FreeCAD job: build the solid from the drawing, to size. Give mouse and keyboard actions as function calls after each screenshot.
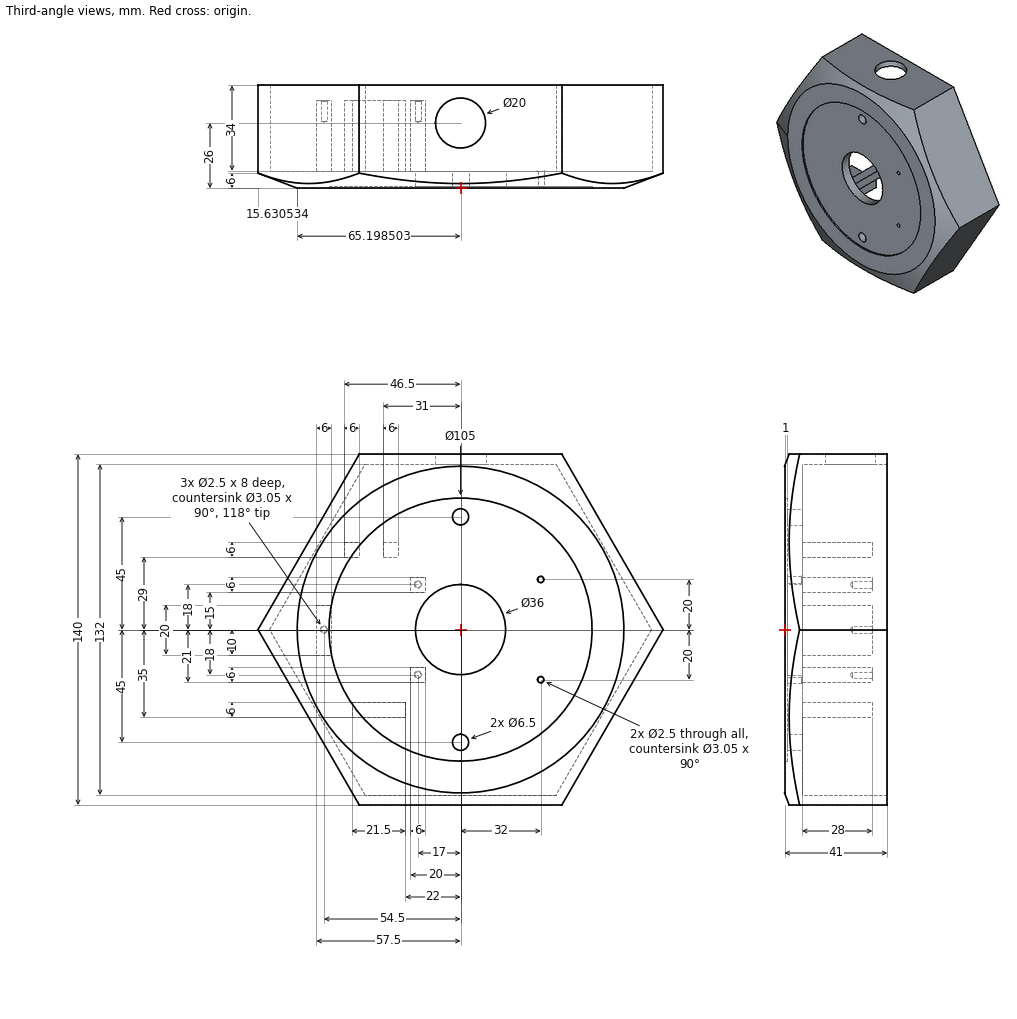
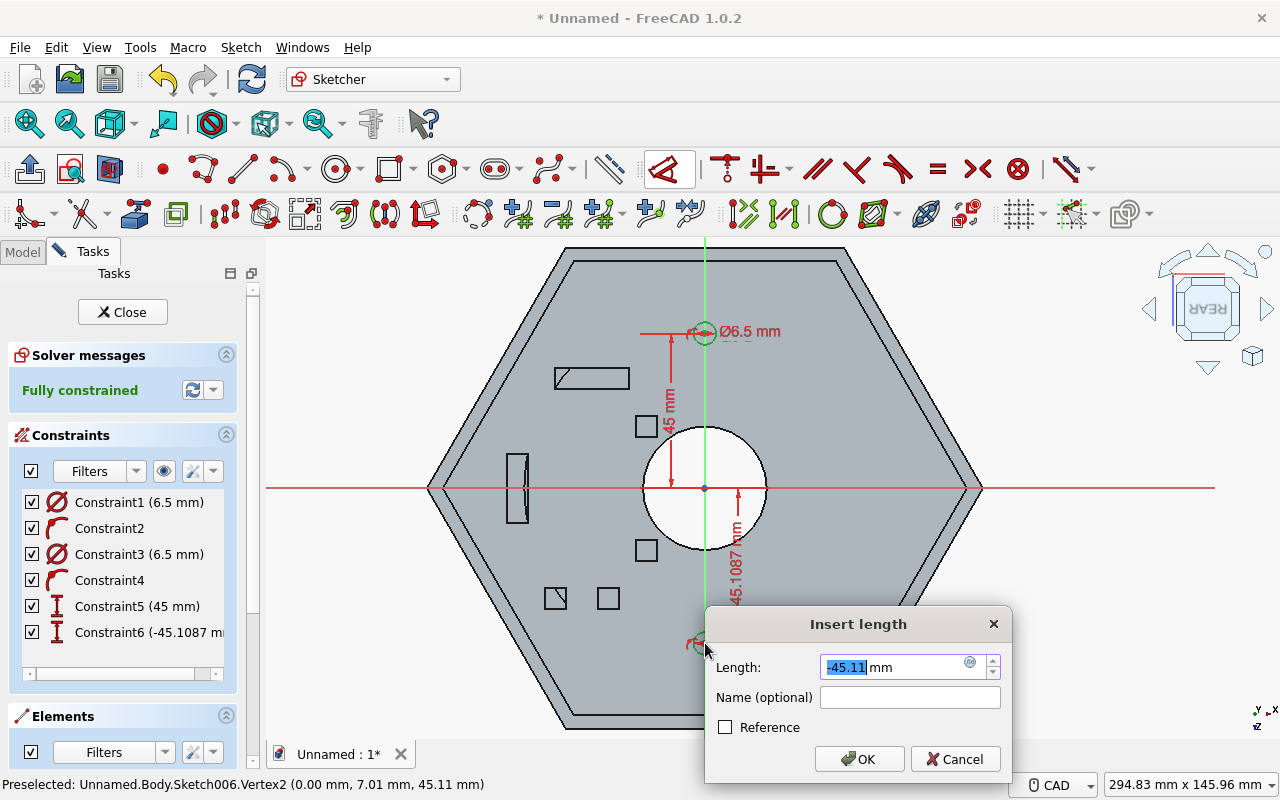
text(-45)
key(Return)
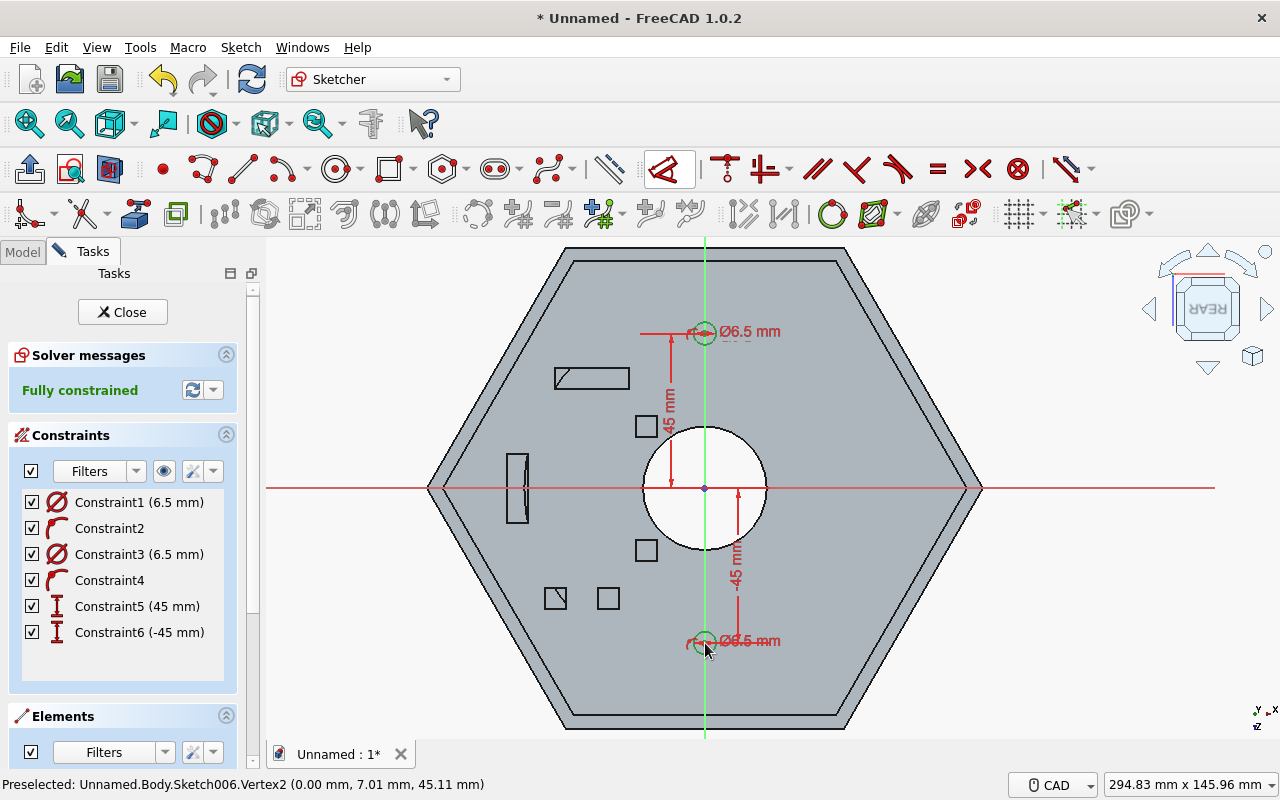
click(123, 312)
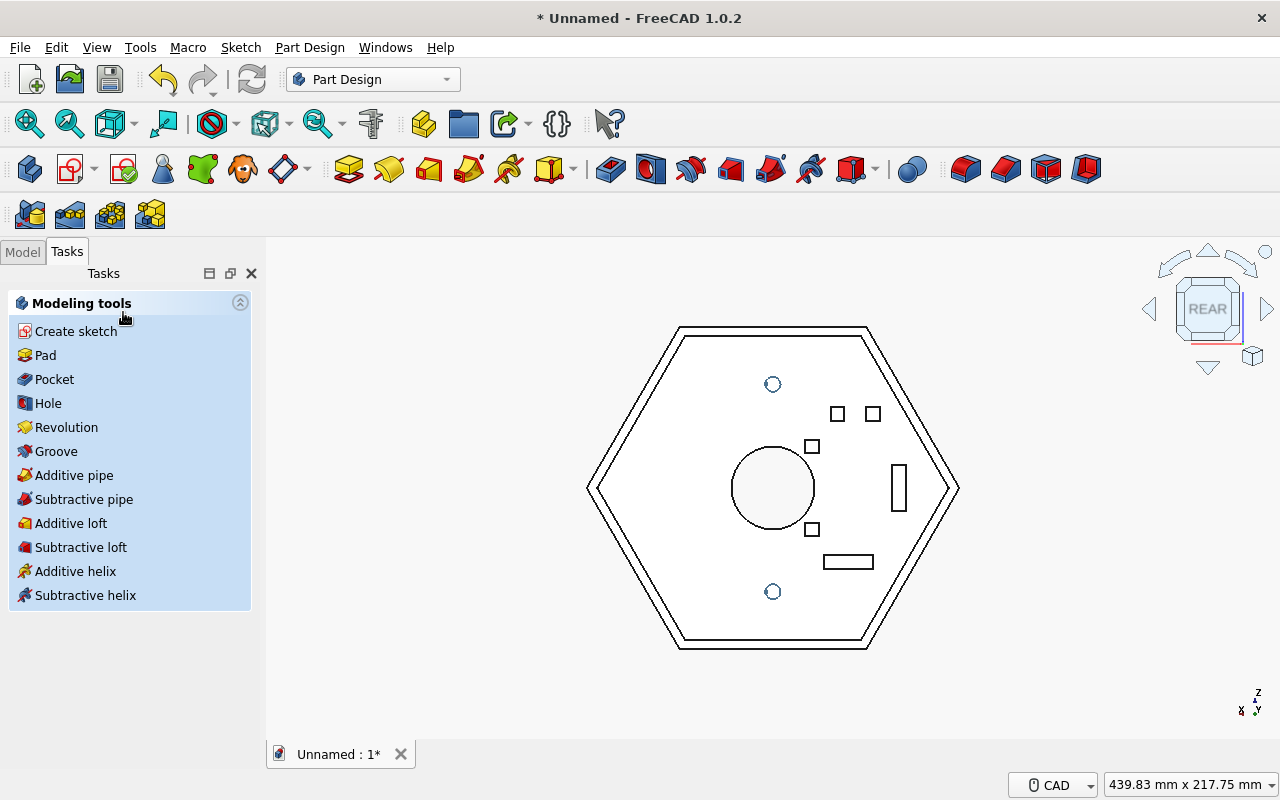
click(612, 170)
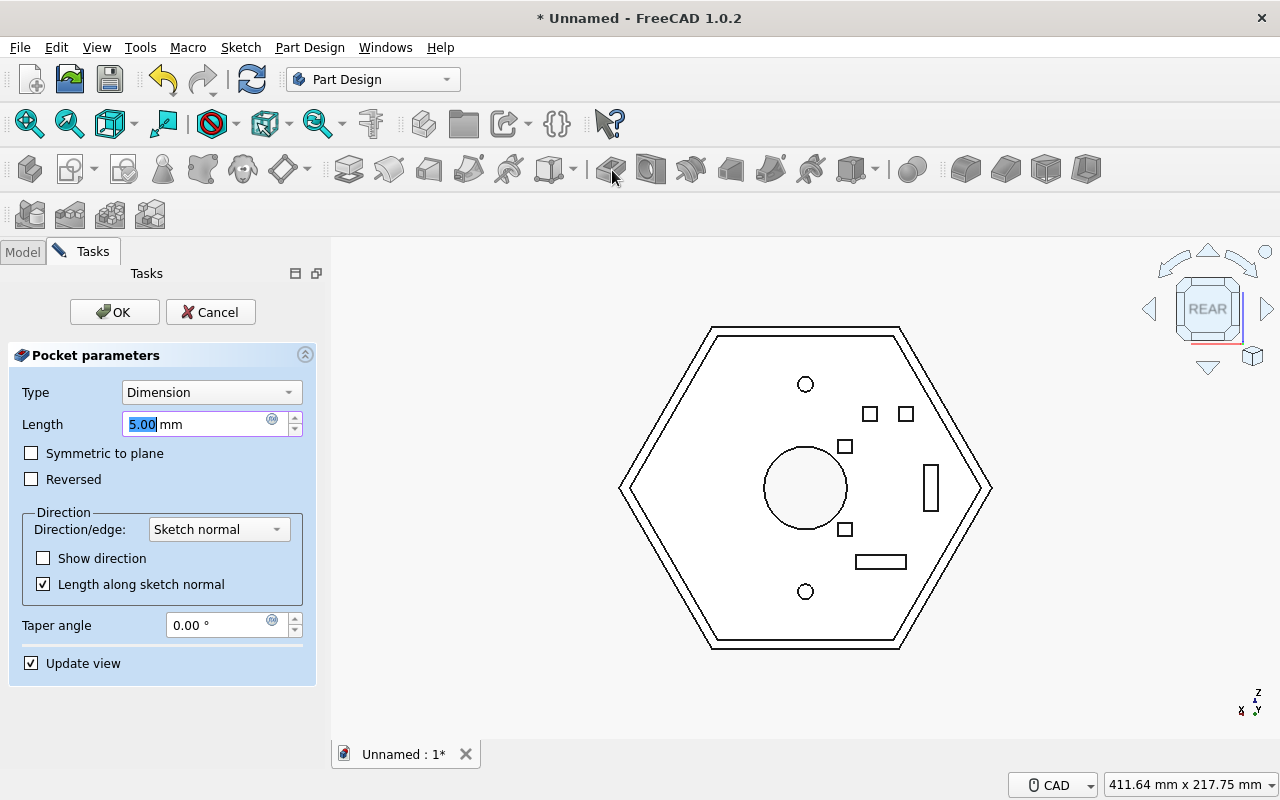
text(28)
key(Tab)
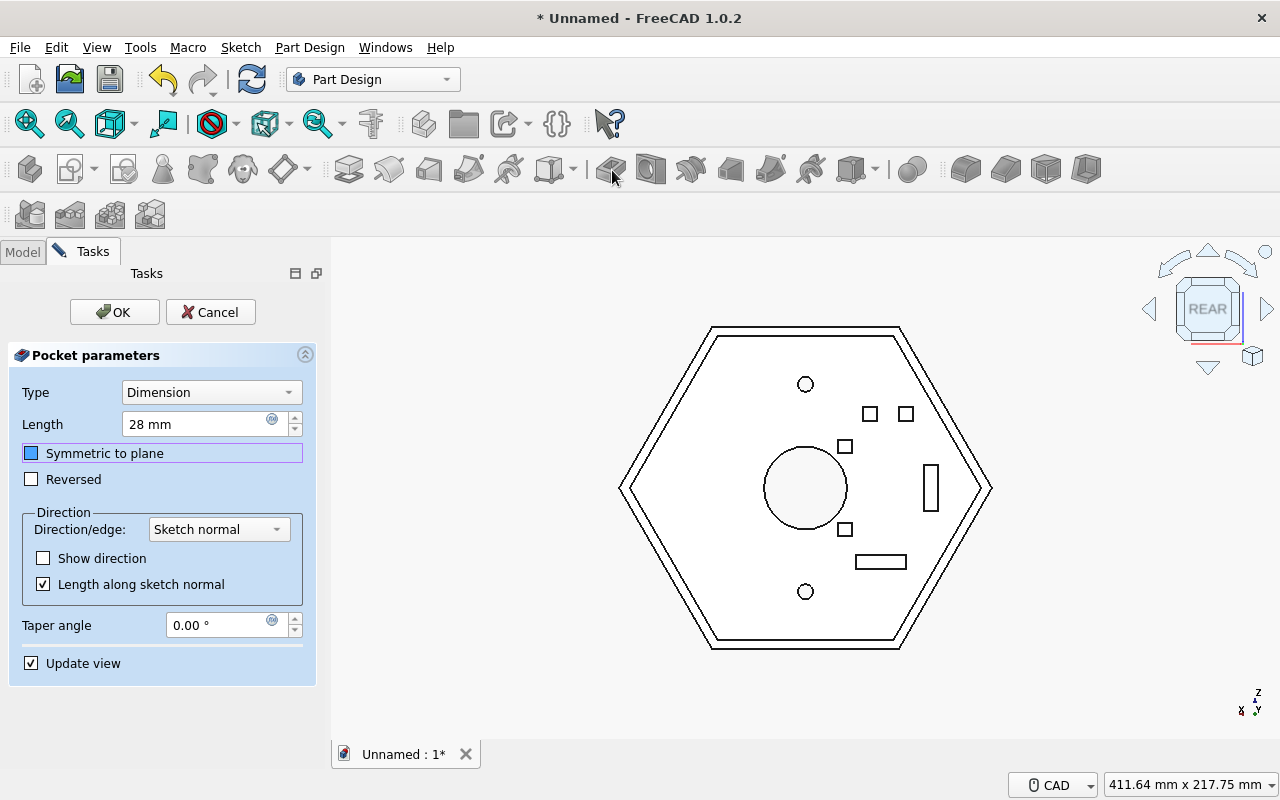
click(115, 312)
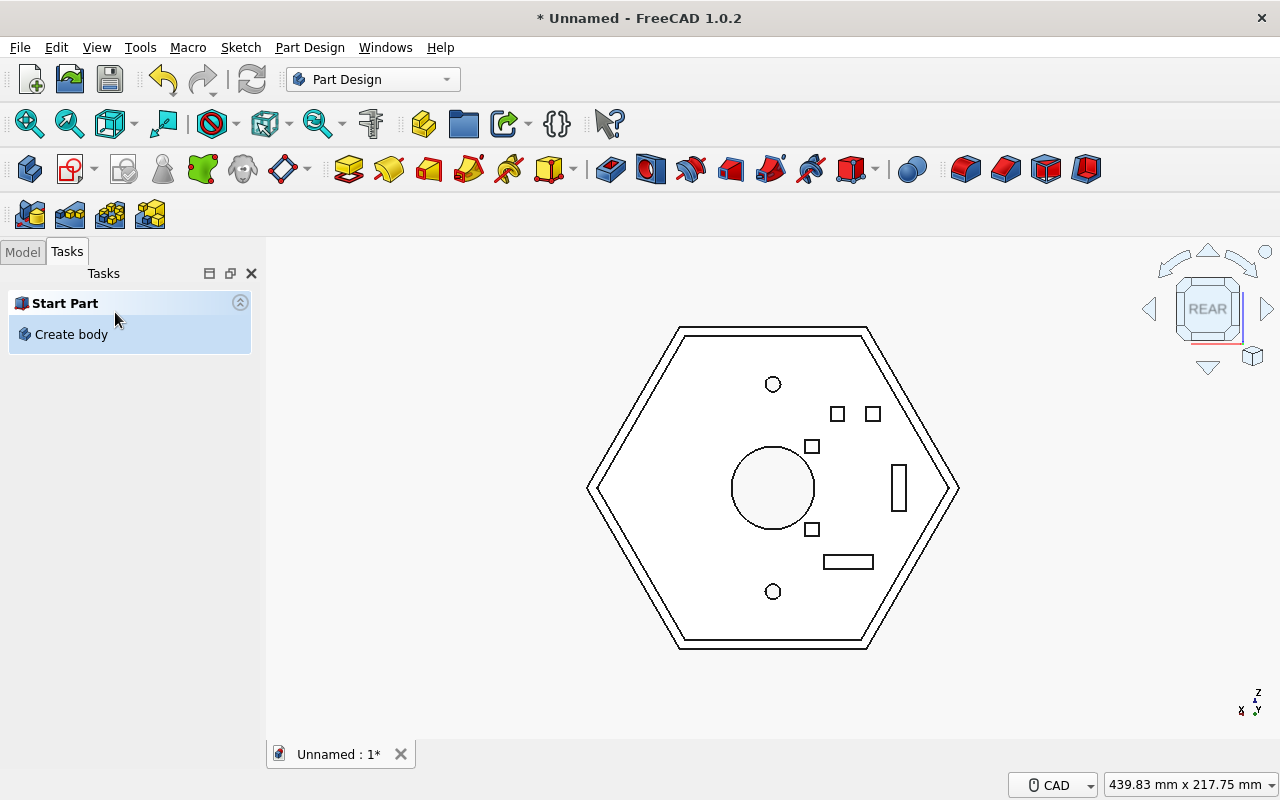
click(673, 487)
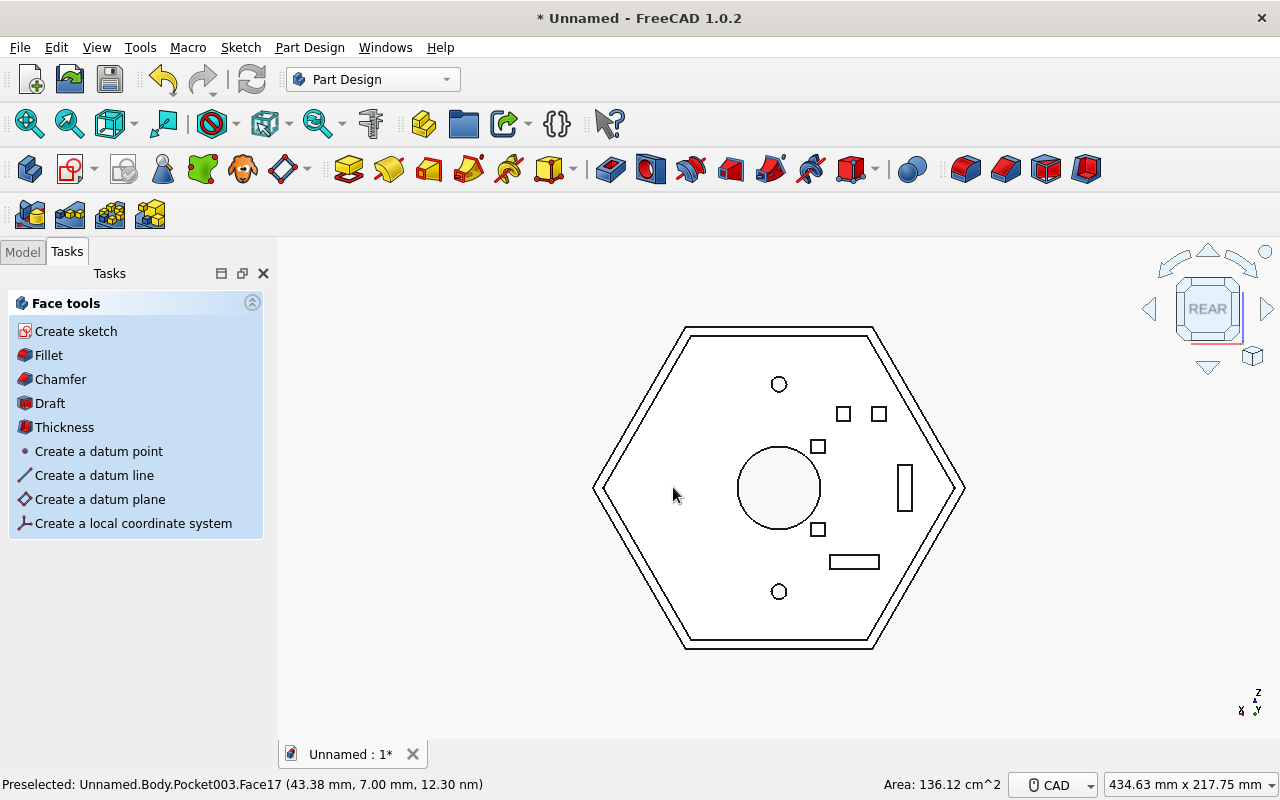
click(70, 170)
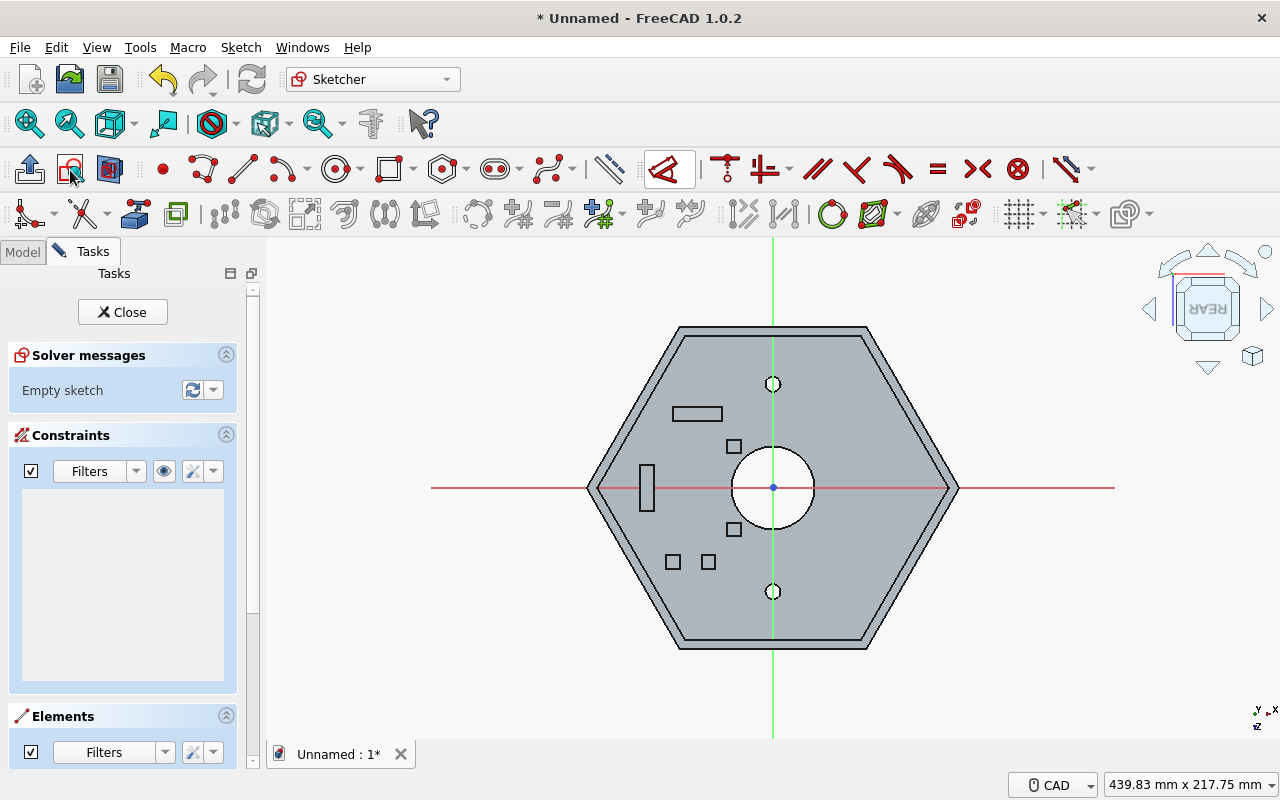
key(q)
key(s)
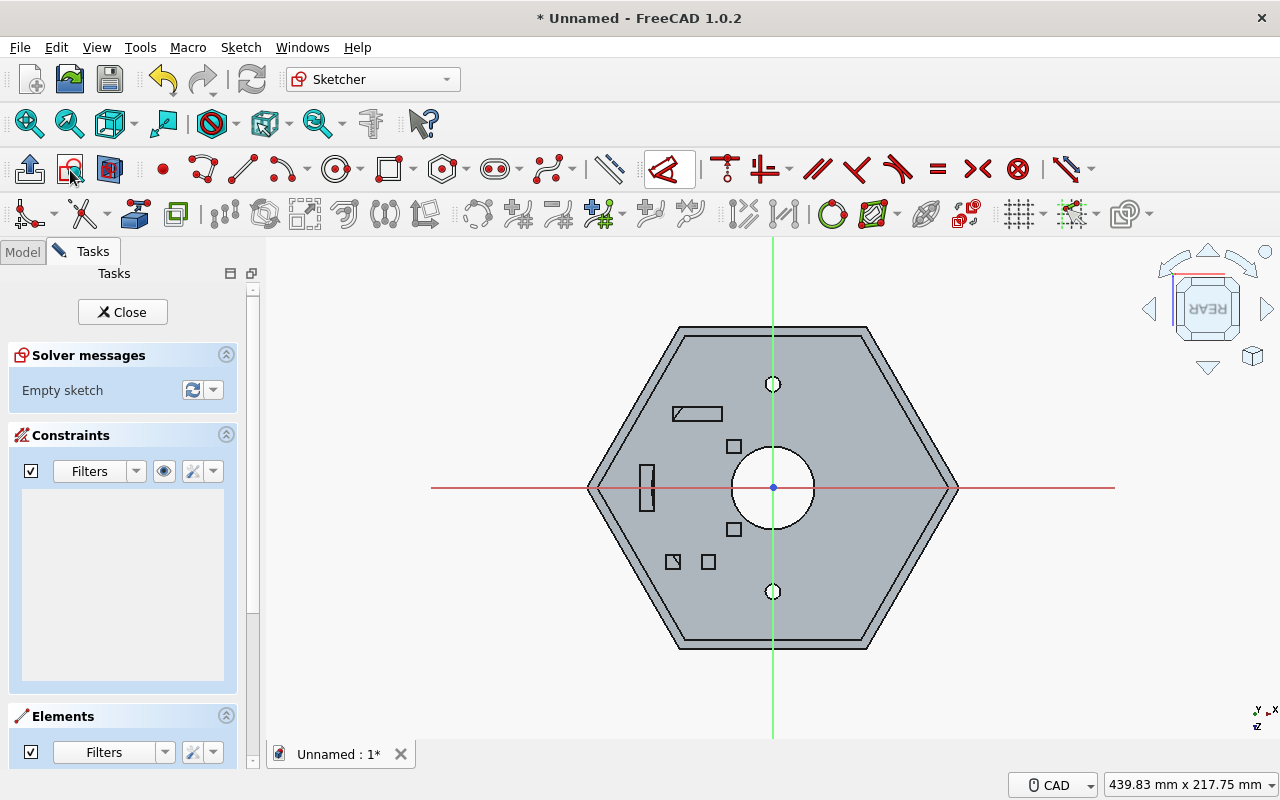
scroll(857, 488, up, 6)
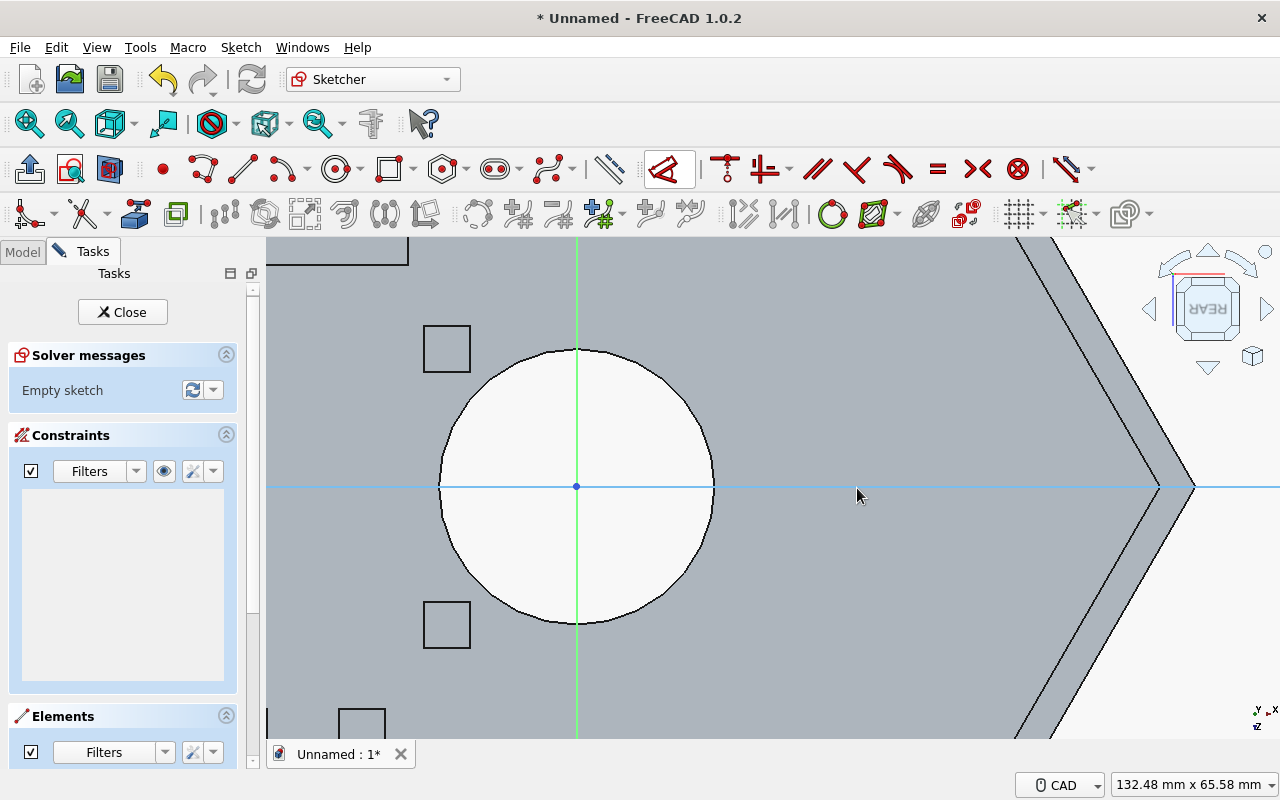
click(336, 170)